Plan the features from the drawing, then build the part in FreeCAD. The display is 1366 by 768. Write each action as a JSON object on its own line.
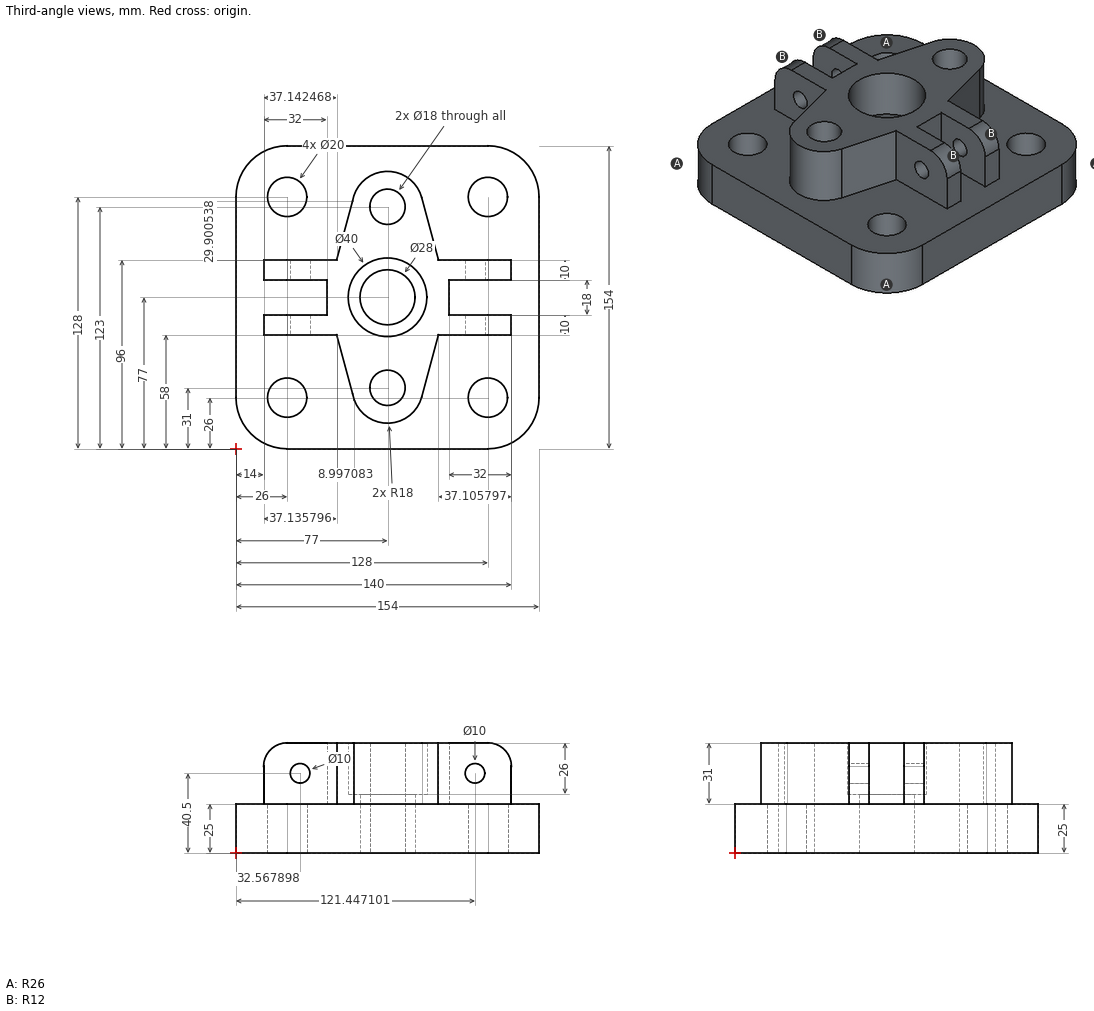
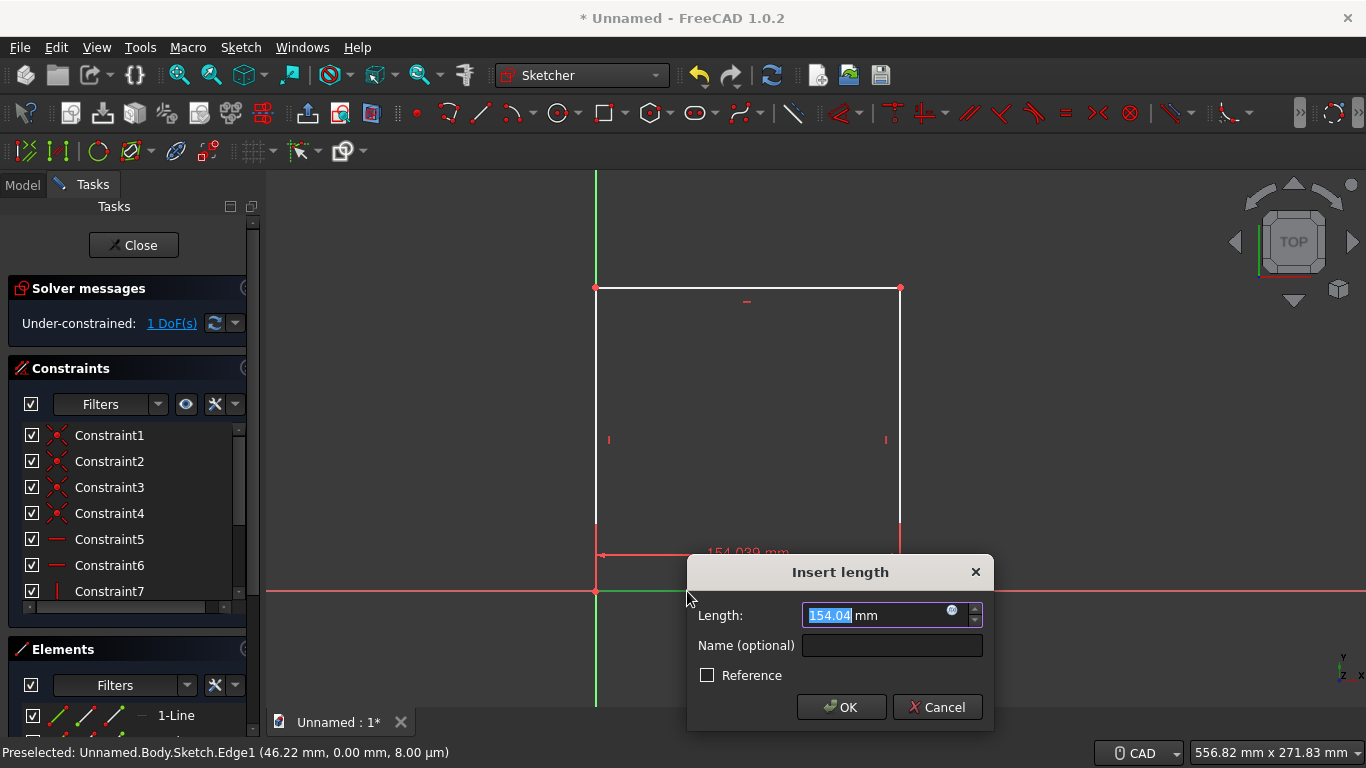
{"action": "type", "text": "154"}
{"action": "key", "text": "Return"}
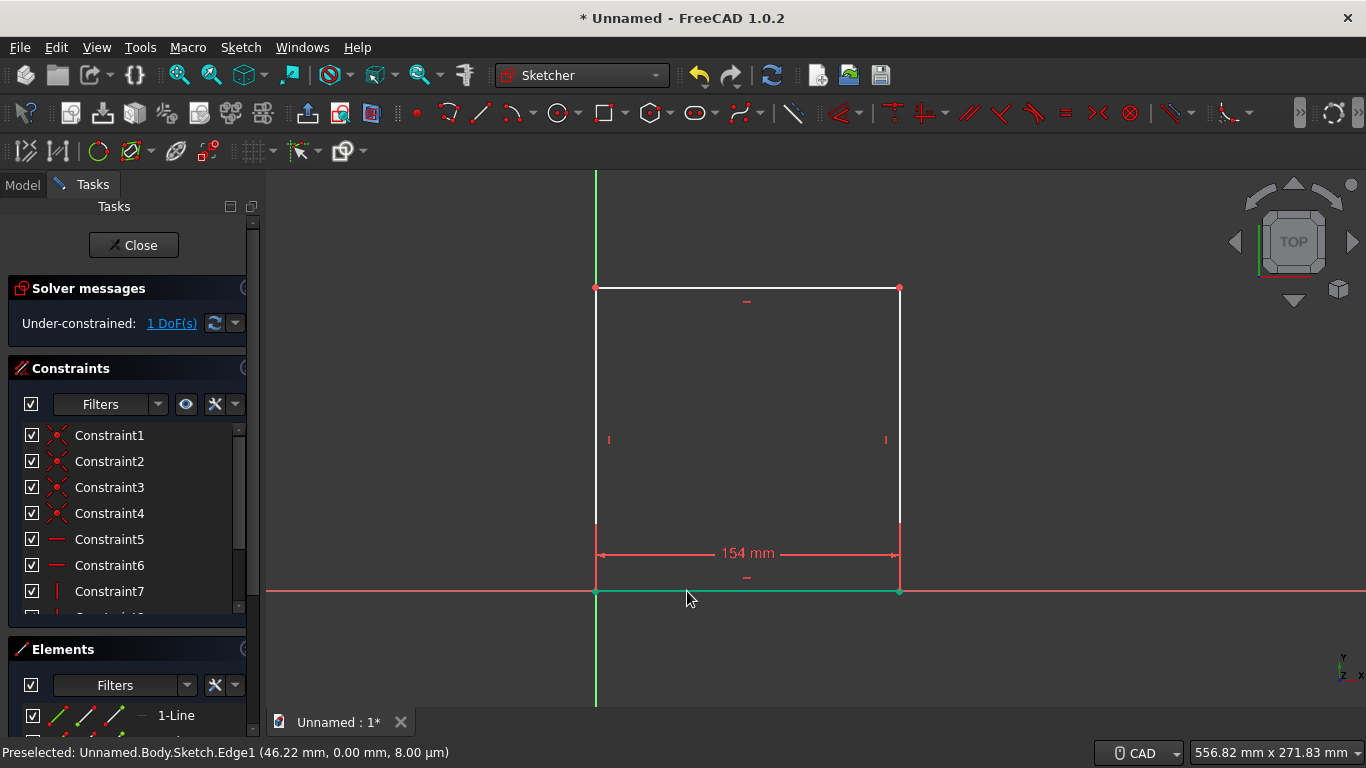
{"action": "left_click", "coordinate": [900, 500]}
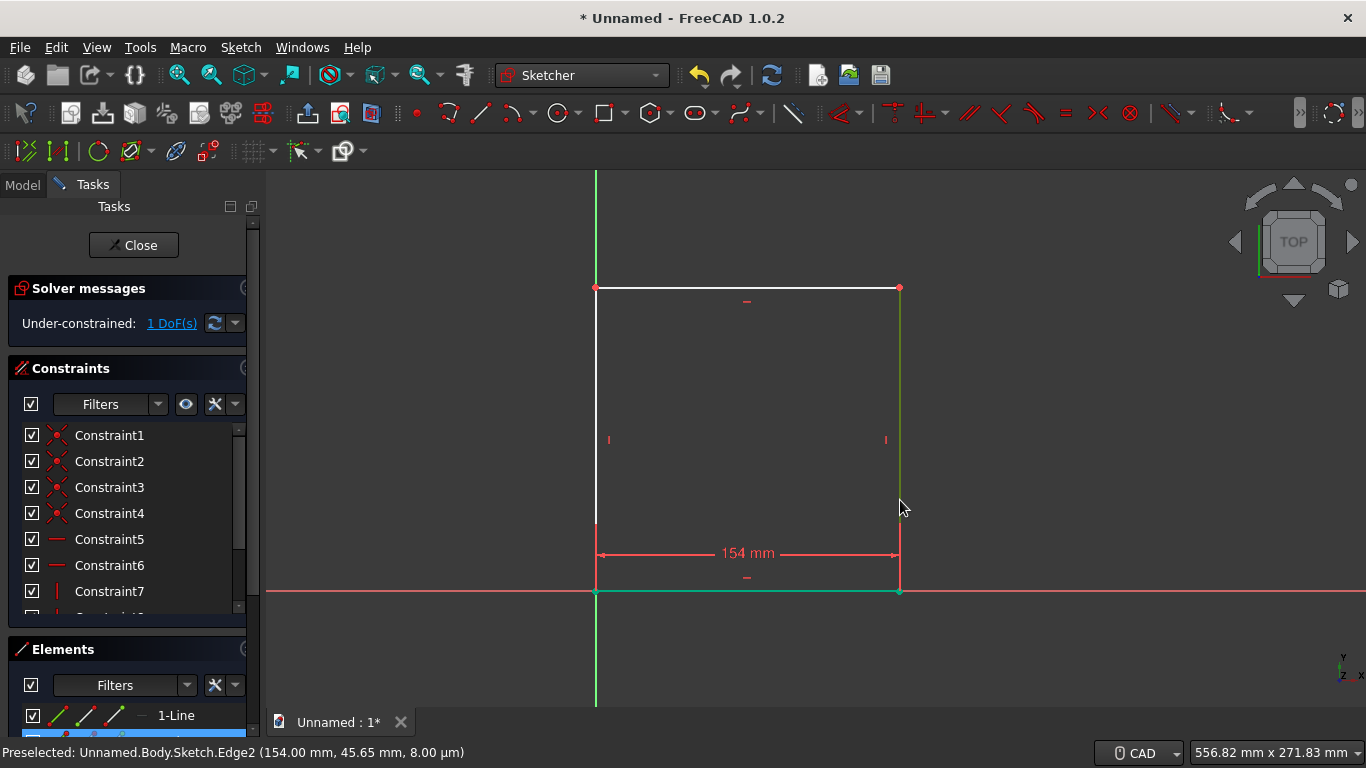
{"action": "left_click", "coordinate": [862, 114]}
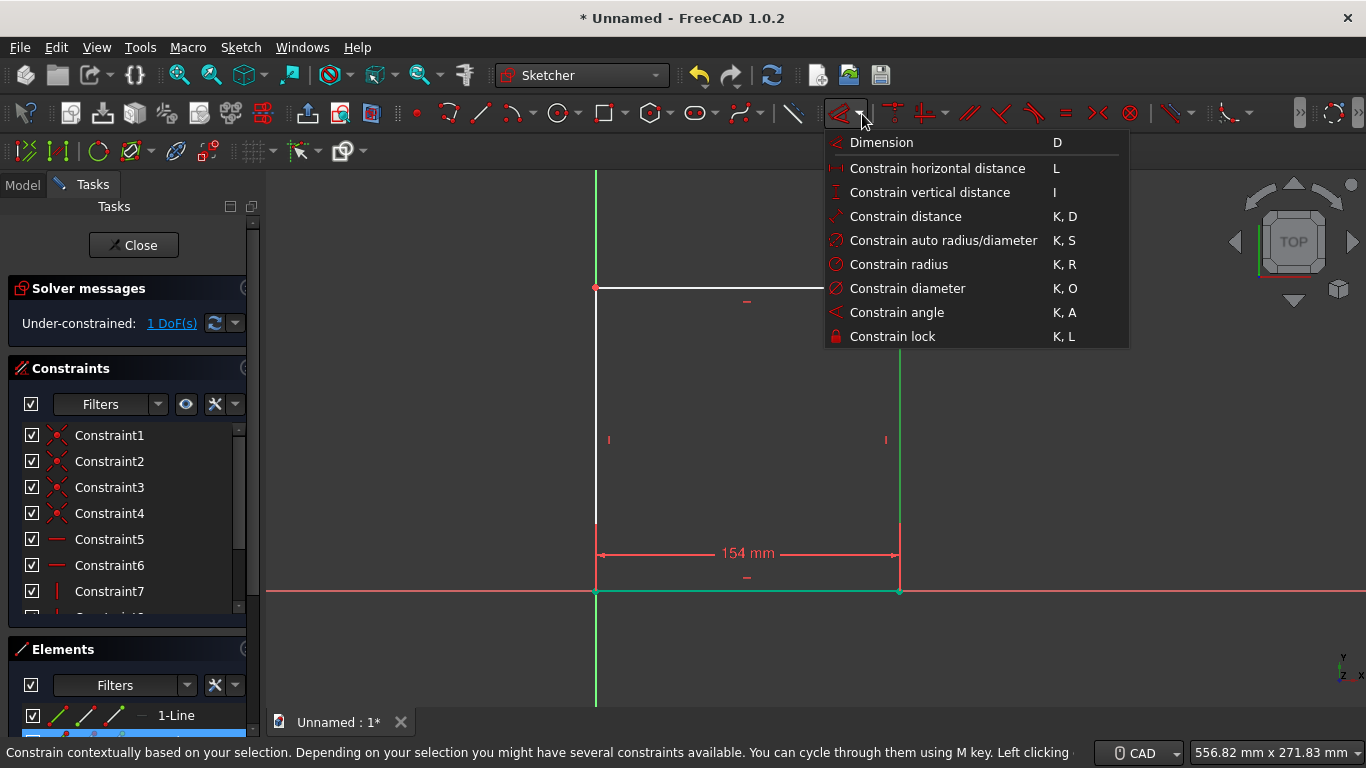
{"action": "left_click", "coordinate": [977, 192]}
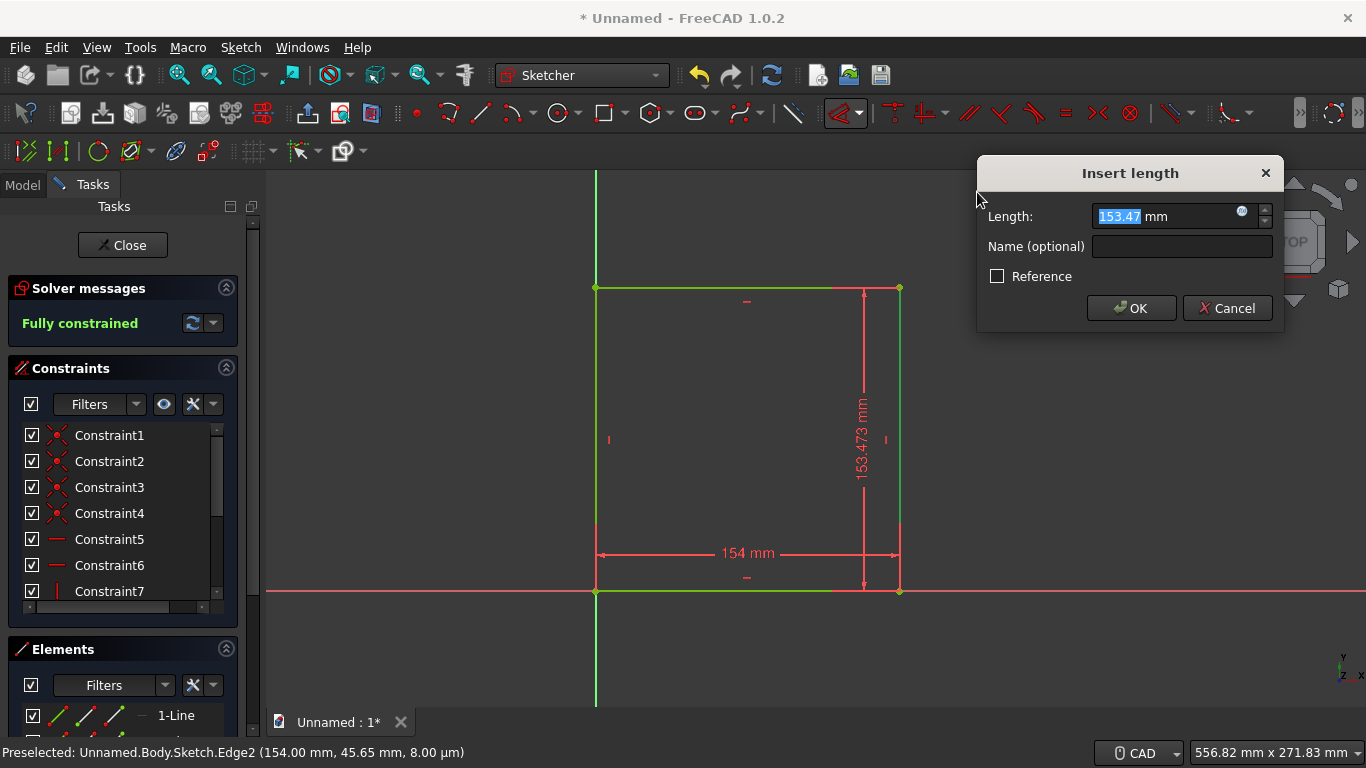
{"action": "type", "text": "154"}
{"action": "key", "text": "Return"}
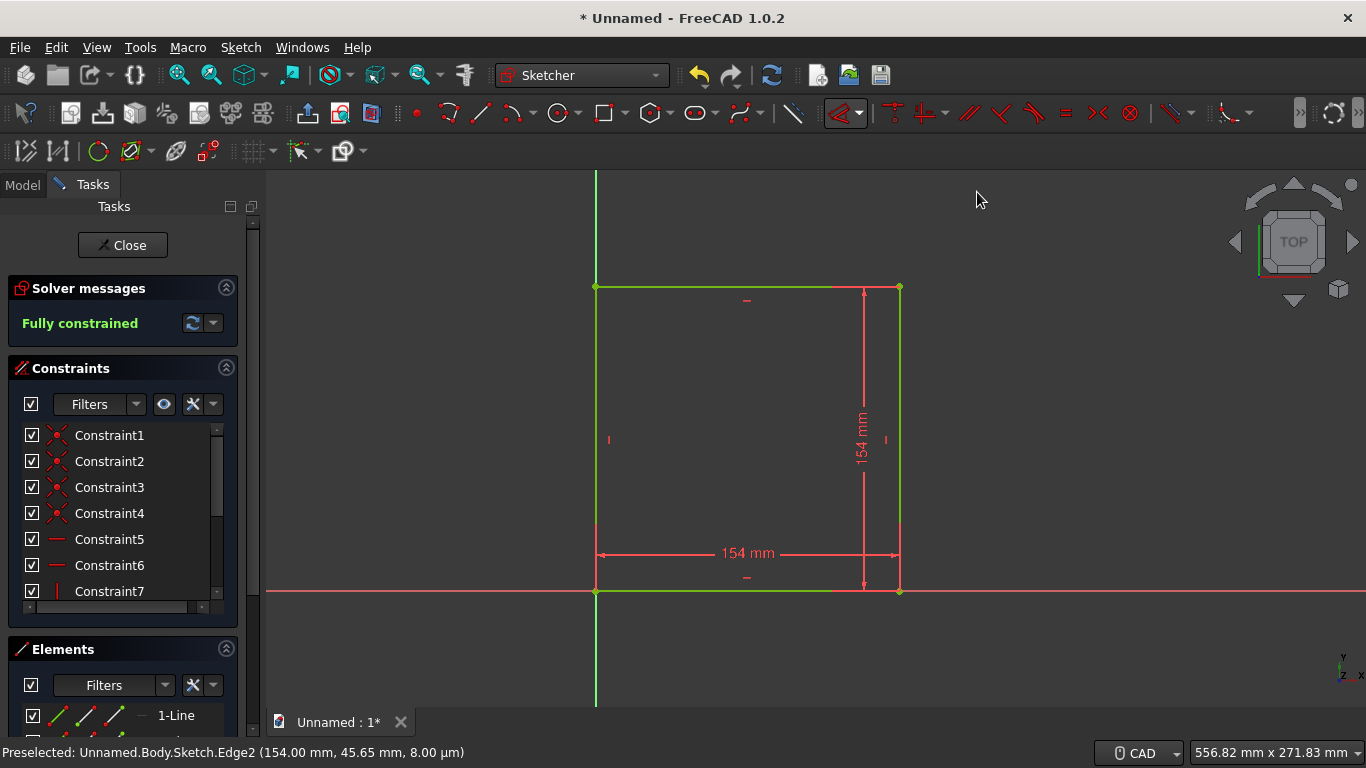
{"action": "left_click", "coordinate": [123, 245]}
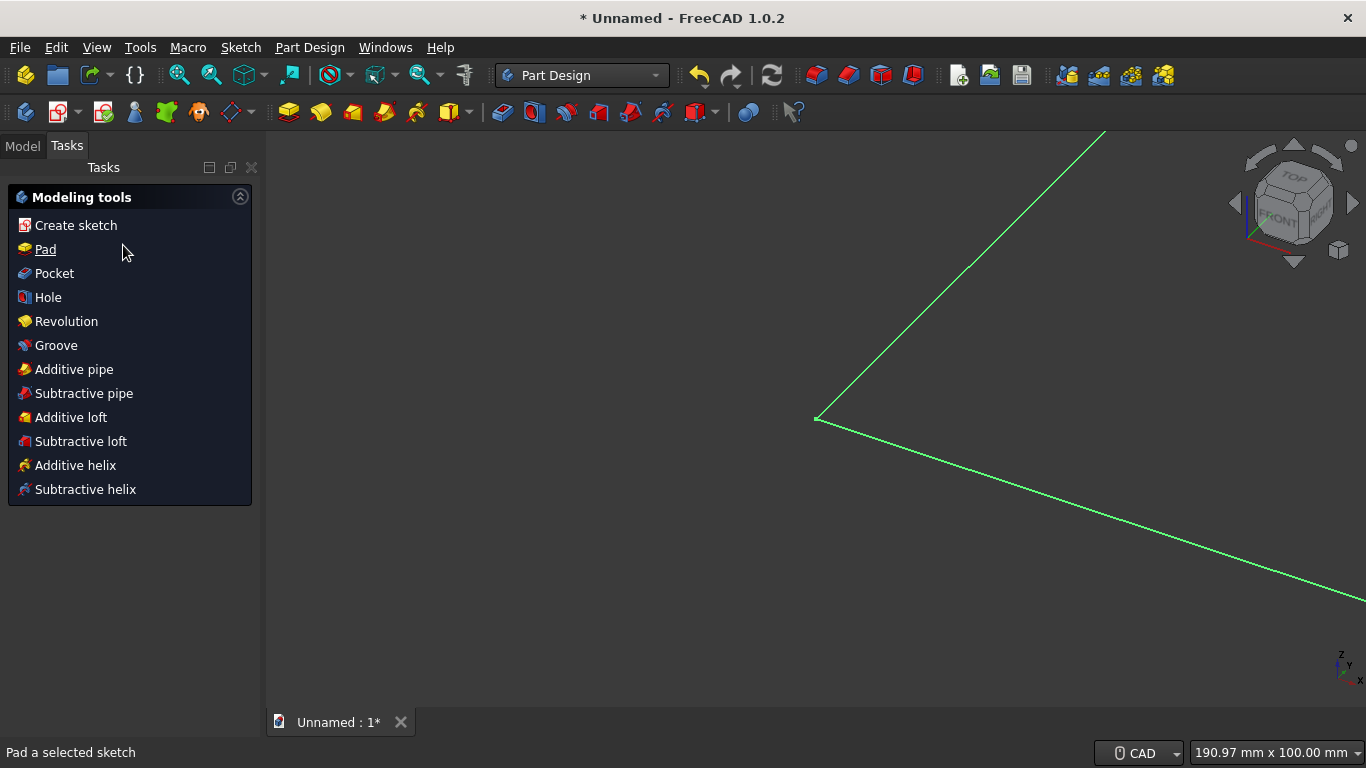
{"action": "left_click", "coordinate": [290, 112]}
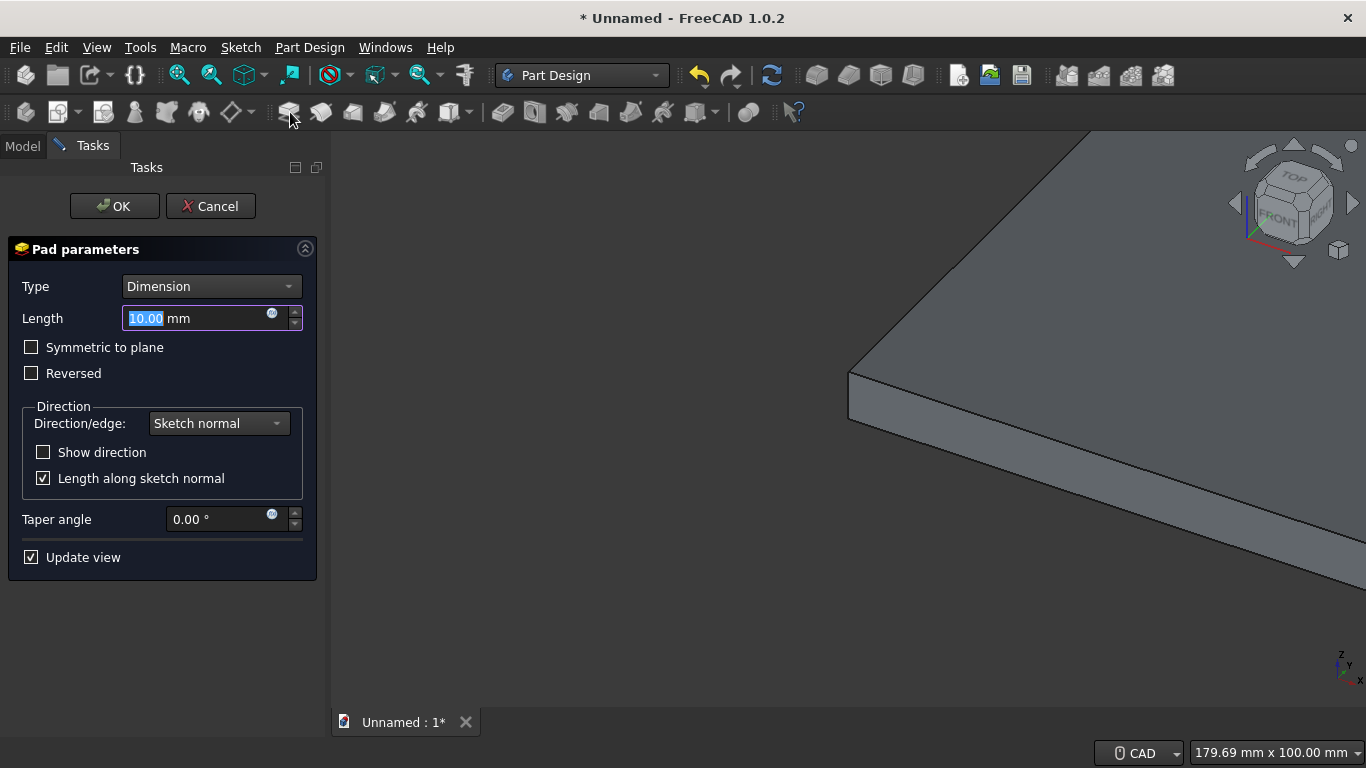
{"action": "type", "text": "25"}
{"action": "key", "text": "Tab"}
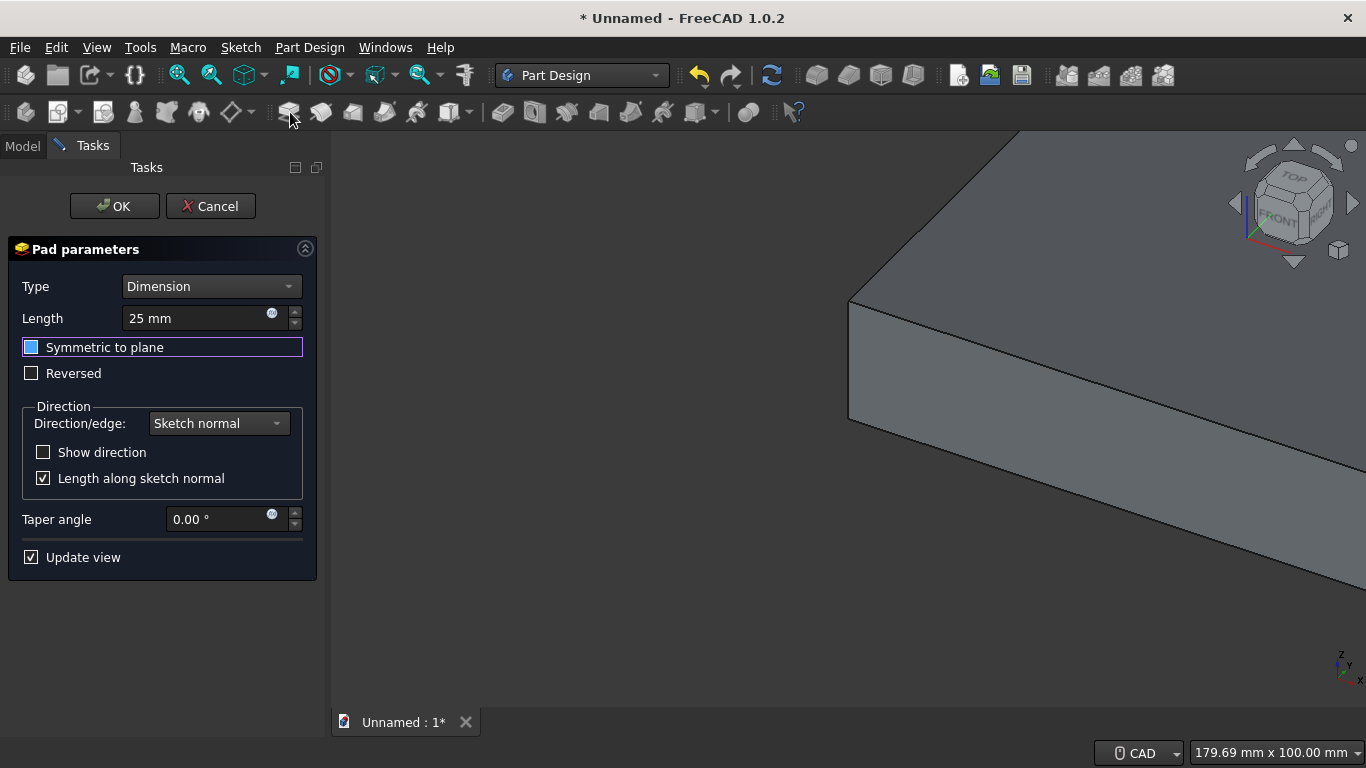
{"action": "left_click", "coordinate": [115, 206]}